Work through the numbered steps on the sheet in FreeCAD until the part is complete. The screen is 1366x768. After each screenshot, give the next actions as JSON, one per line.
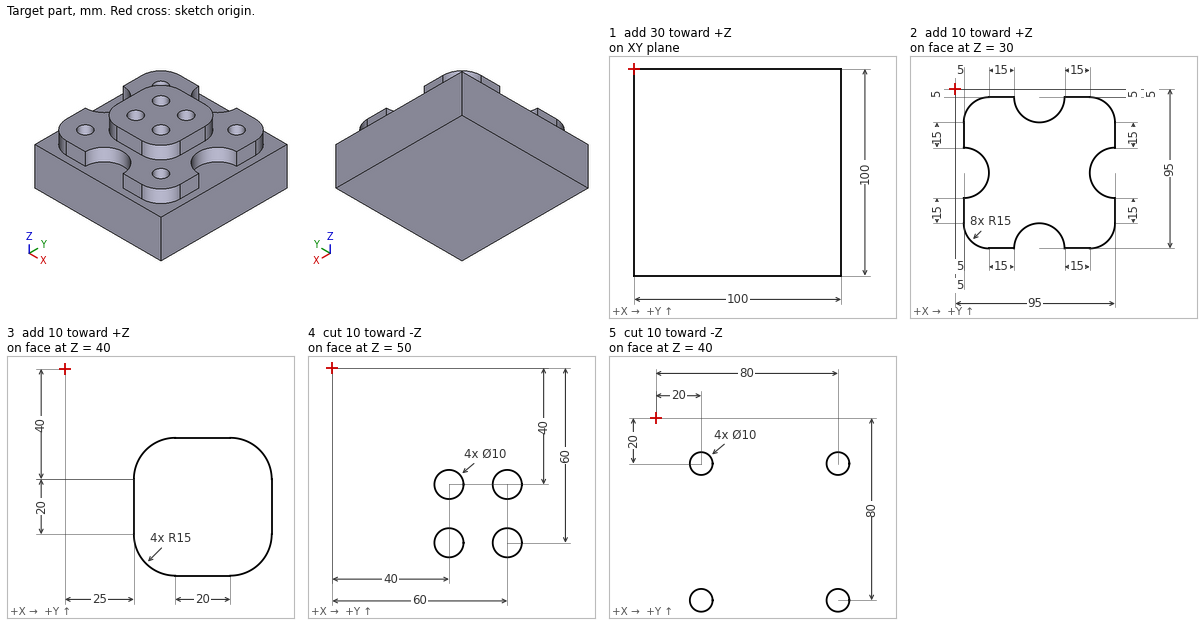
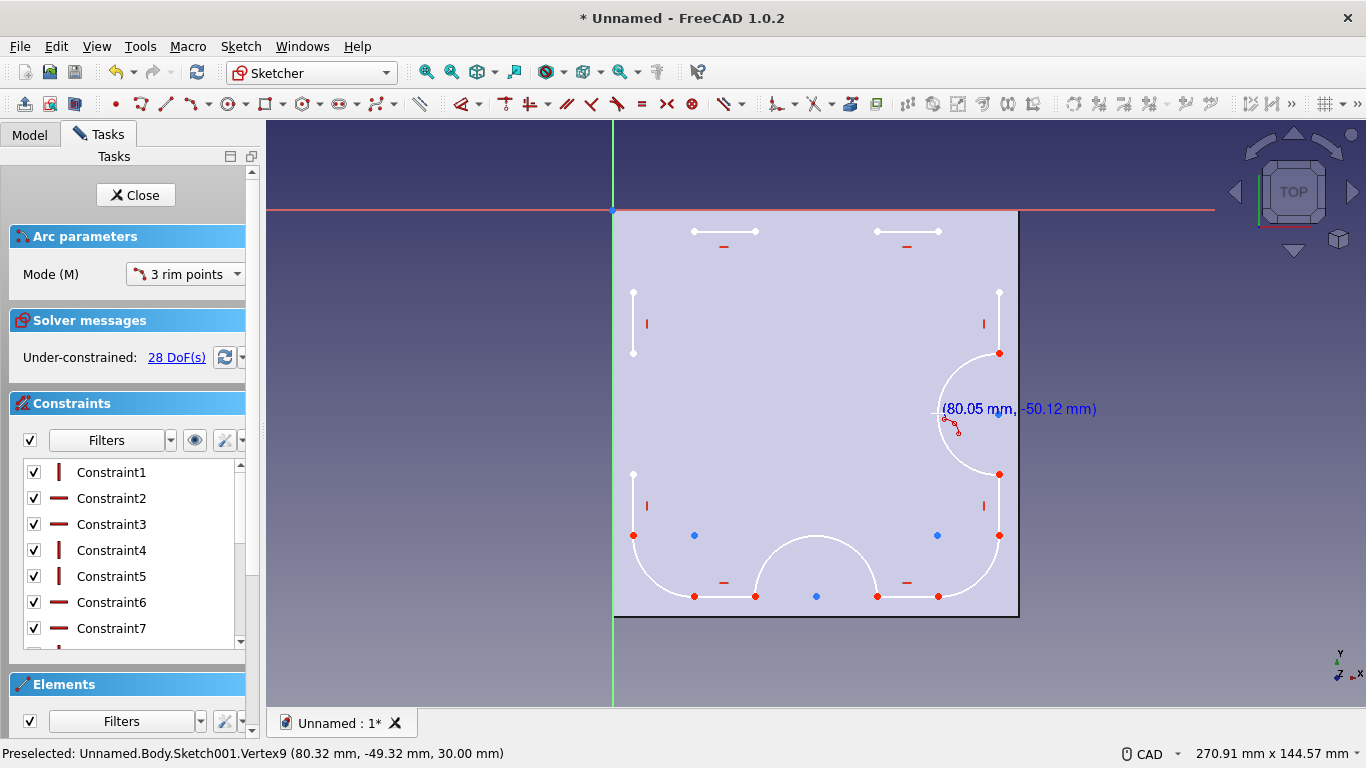
{"action": "left_click", "coordinate": [999, 293]}
{"action": "left_click", "coordinate": [938, 232]}
{"action": "left_click", "coordinate": [981, 249]}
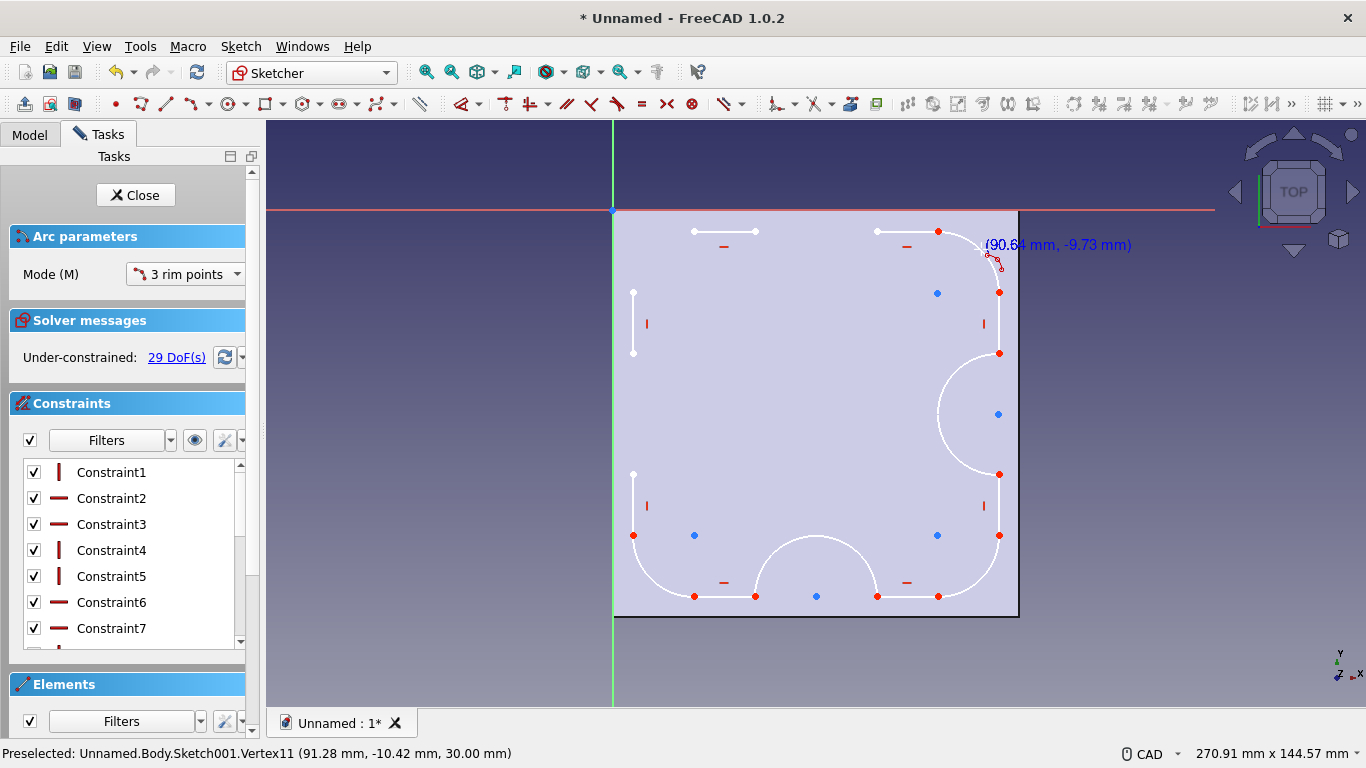
{"action": "left_click", "coordinate": [877, 232]}
{"action": "left_click", "coordinate": [755, 232]}
{"action": "left_click", "coordinate": [816, 292]}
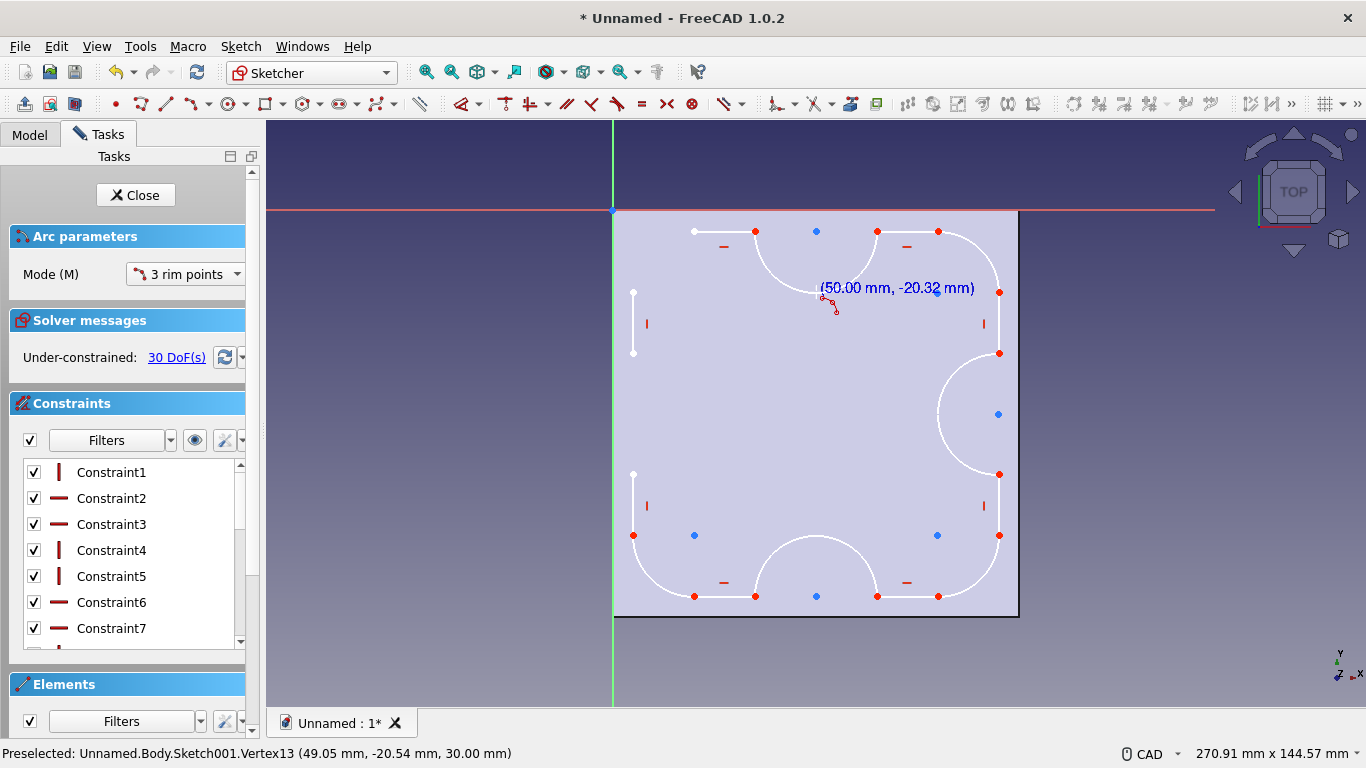
{"action": "left_click", "coordinate": [694, 232]}
{"action": "left_click", "coordinate": [633, 293]}
{"action": "left_click", "coordinate": [651, 249]}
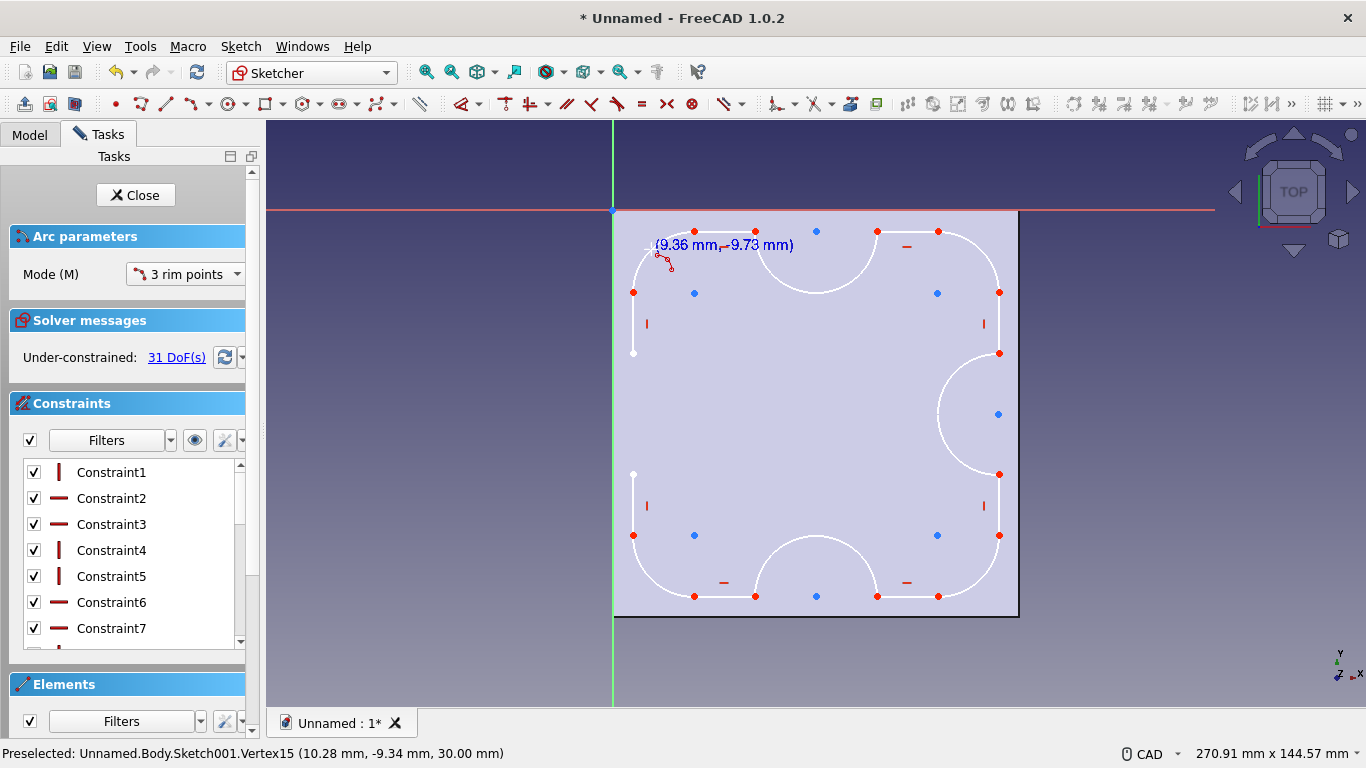
{"action": "left_click", "coordinate": [633, 354]}
{"action": "left_click", "coordinate": [633, 475]}
{"action": "left_click", "coordinate": [694, 413]}
{"action": "key", "text": "Escape"}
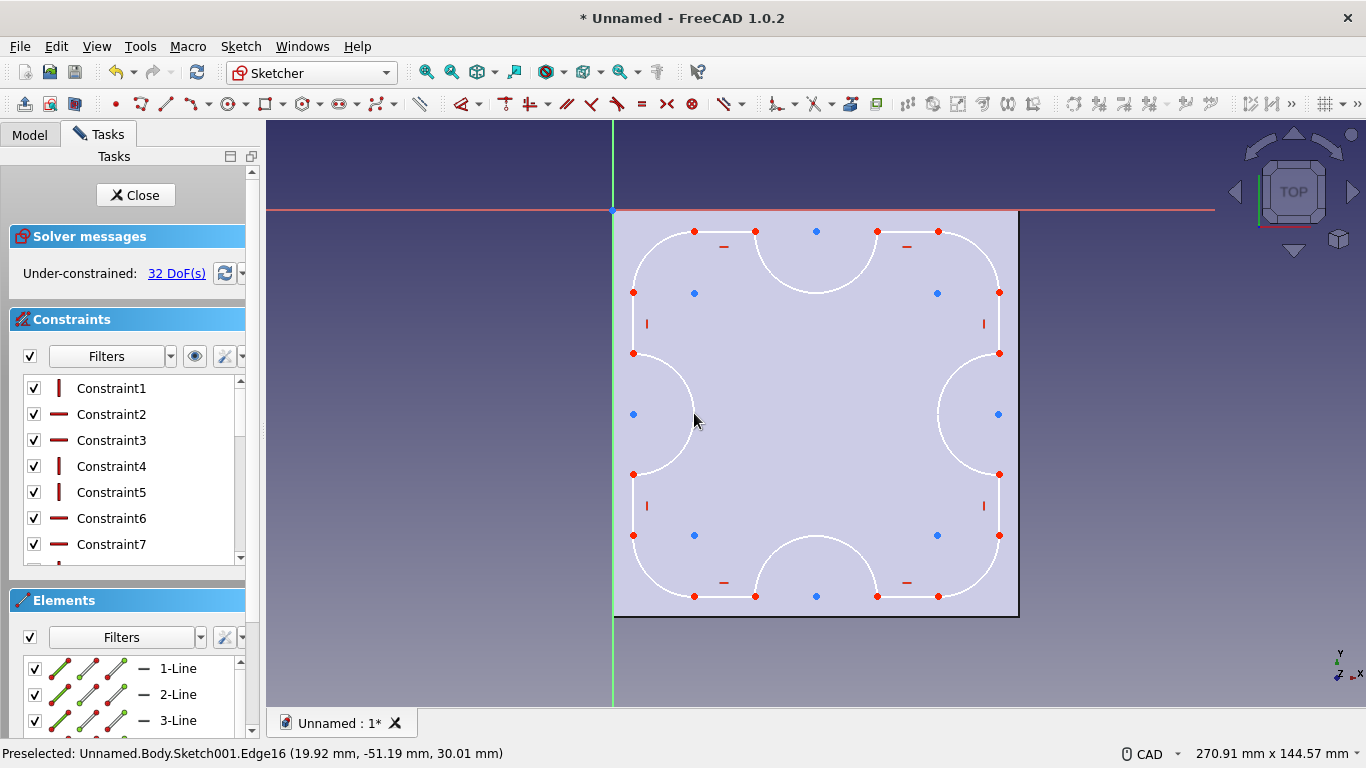
{"action": "left_click", "coordinate": [633, 493]}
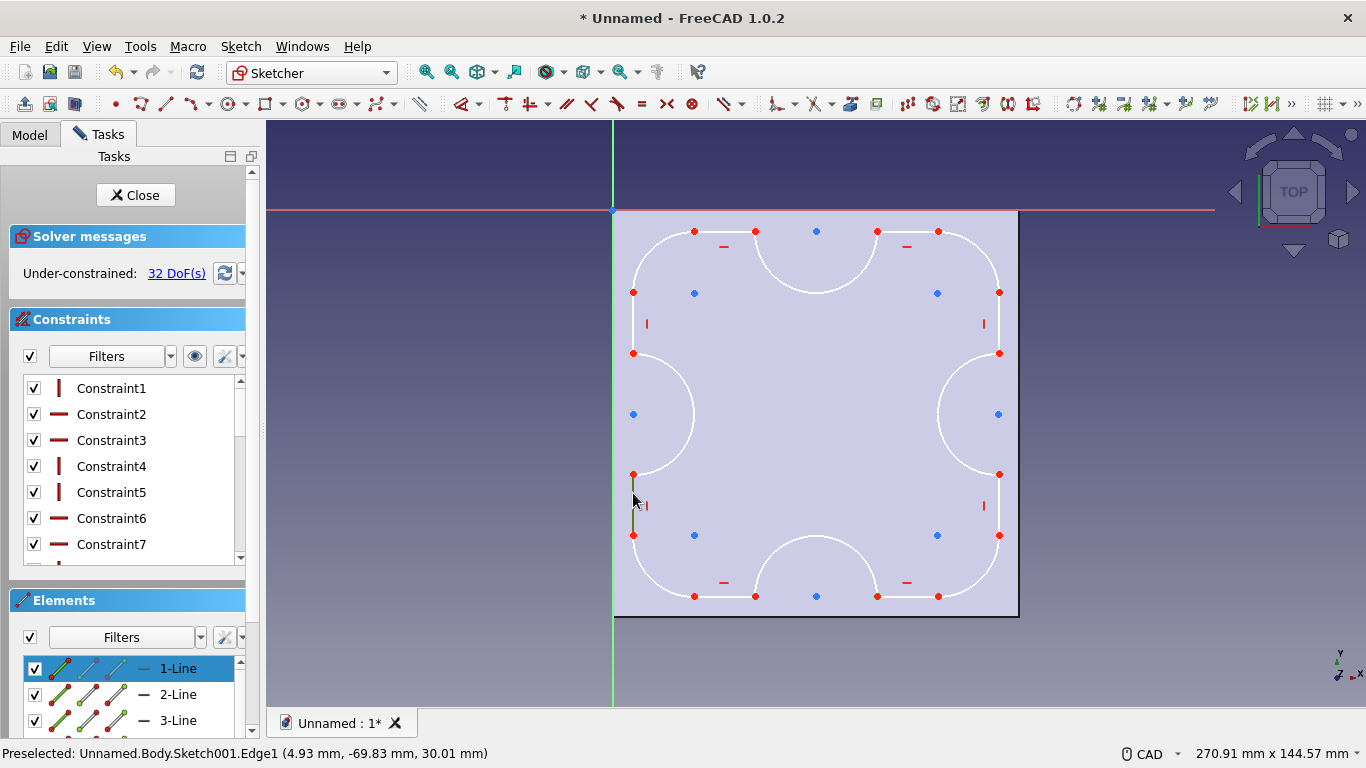
{"action": "left_click", "coordinate": [640, 564]}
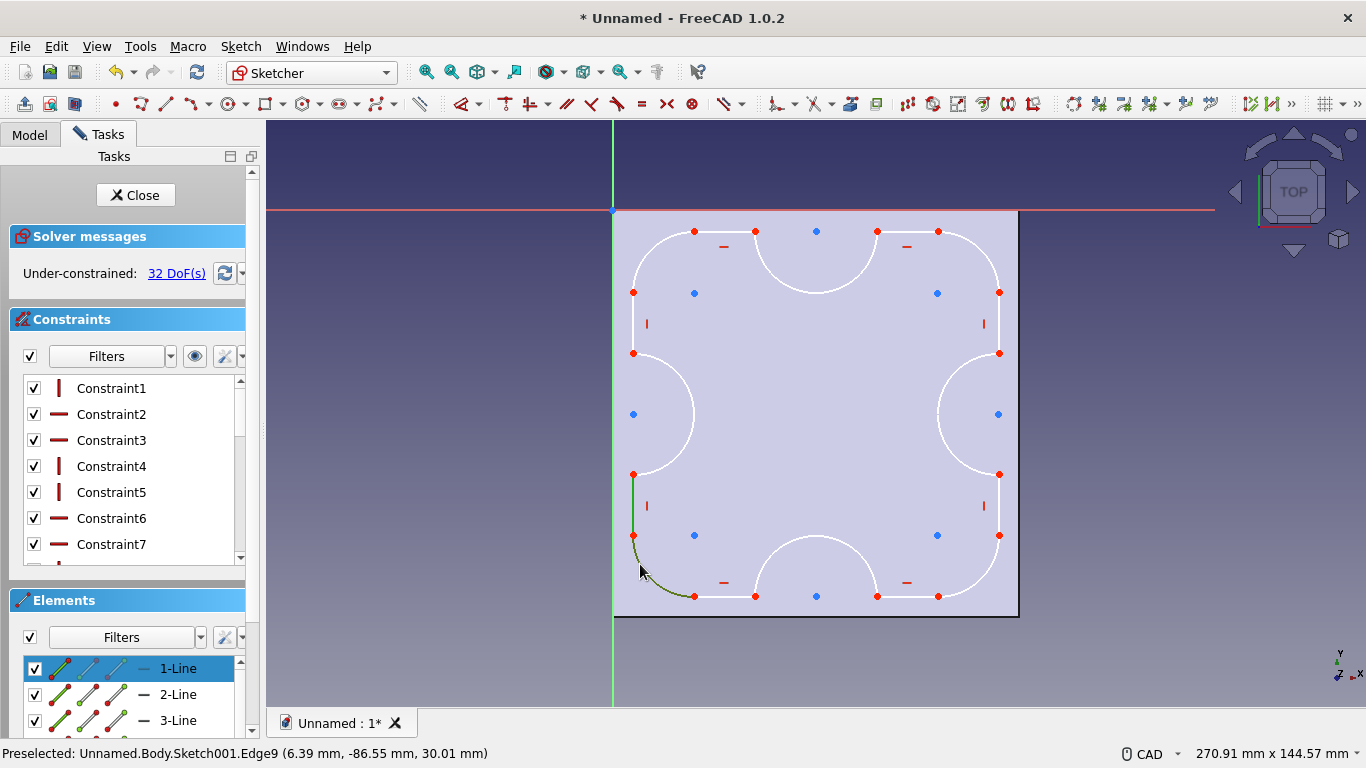
{"action": "key", "text": "t"}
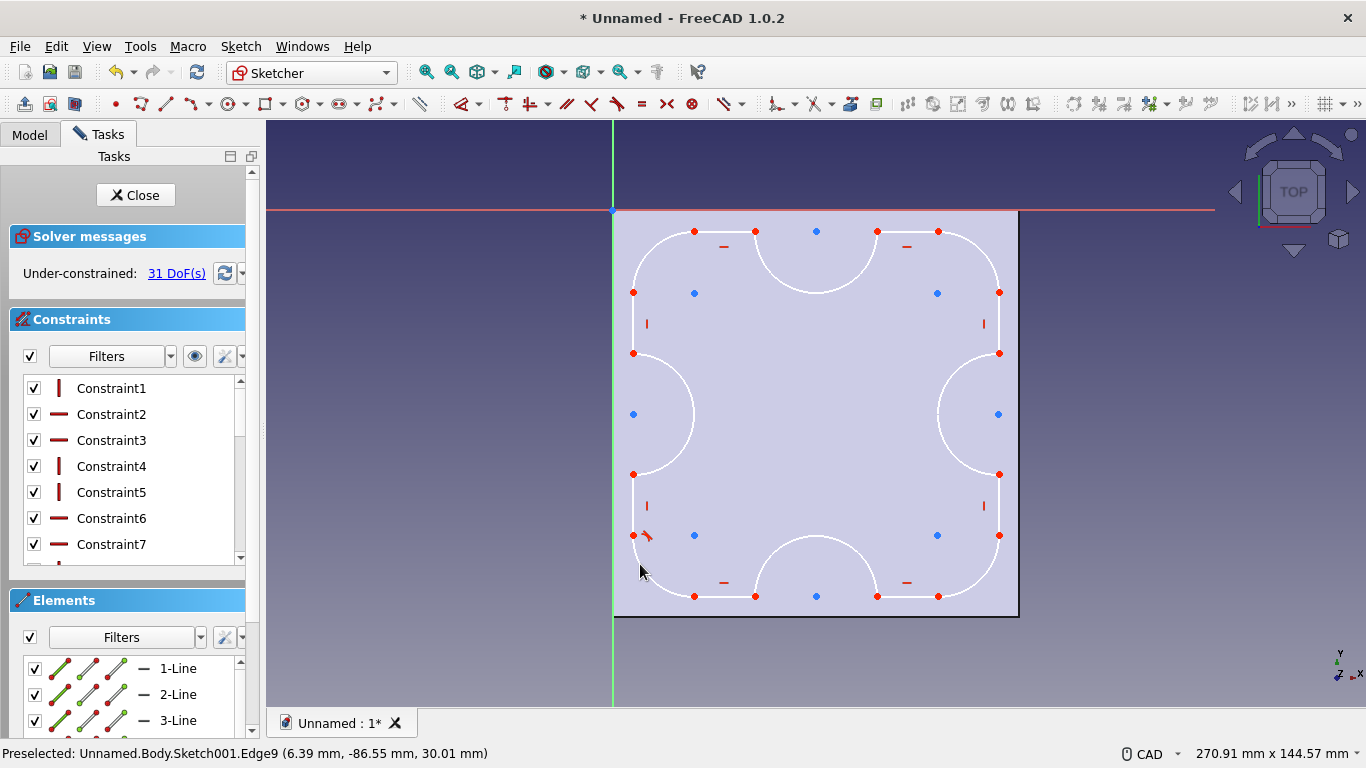
{"action": "left_click", "coordinate": [712, 597]}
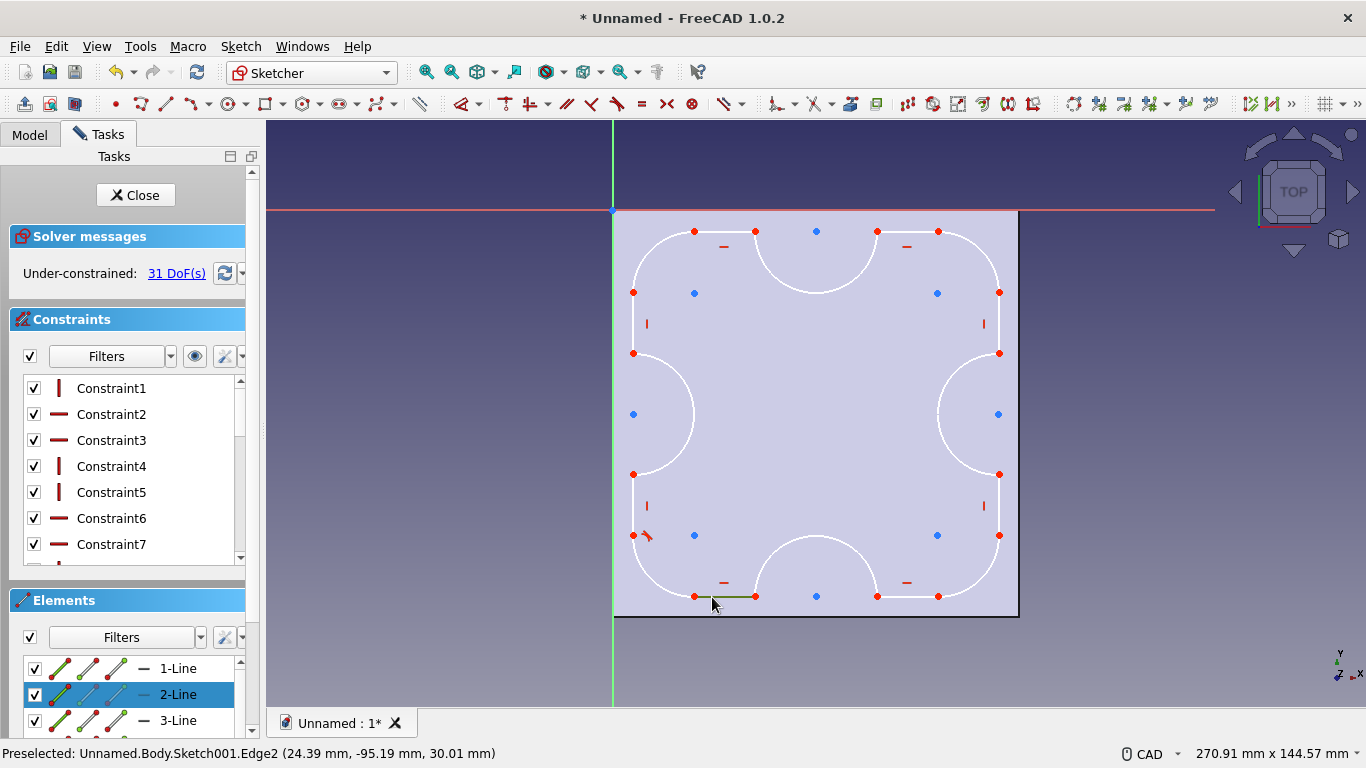
{"action": "left_click", "coordinate": [640, 563]}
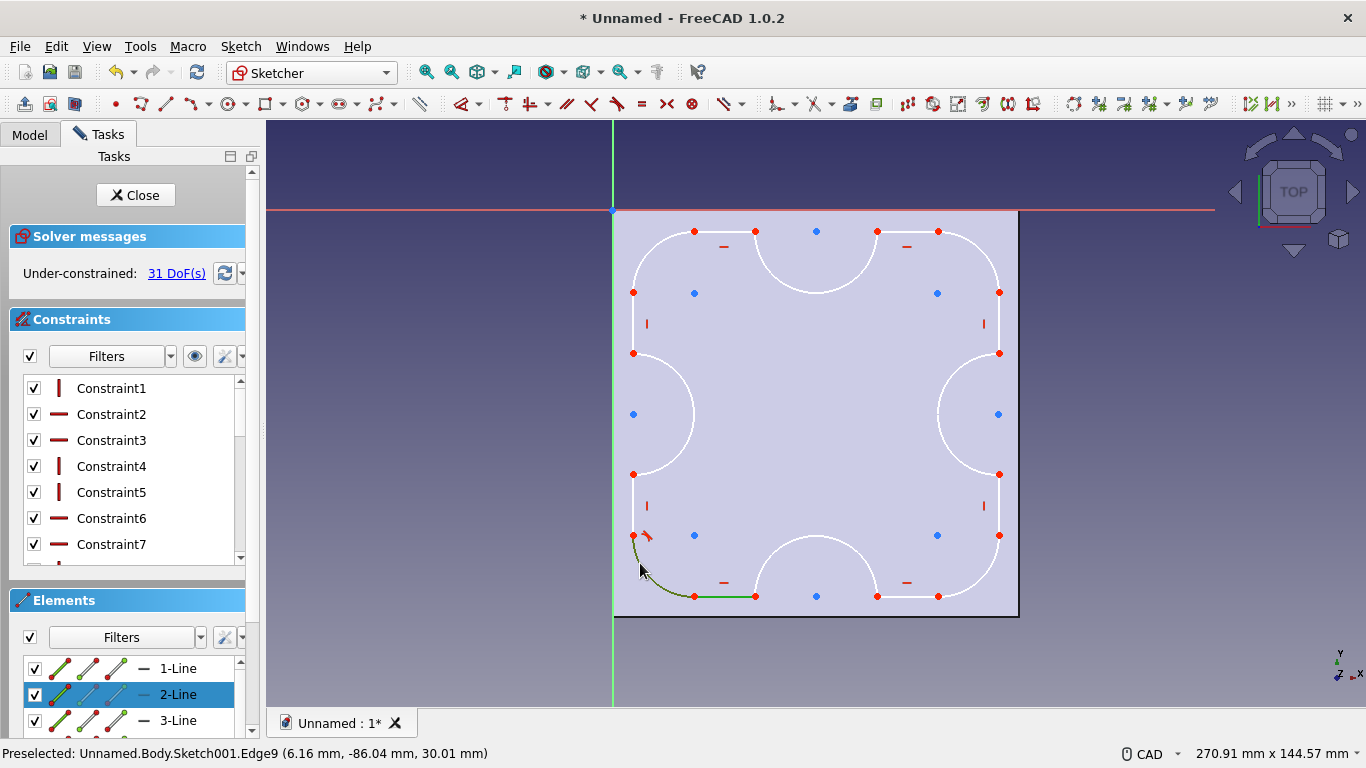
{"action": "left_click", "coordinate": [617, 104]}